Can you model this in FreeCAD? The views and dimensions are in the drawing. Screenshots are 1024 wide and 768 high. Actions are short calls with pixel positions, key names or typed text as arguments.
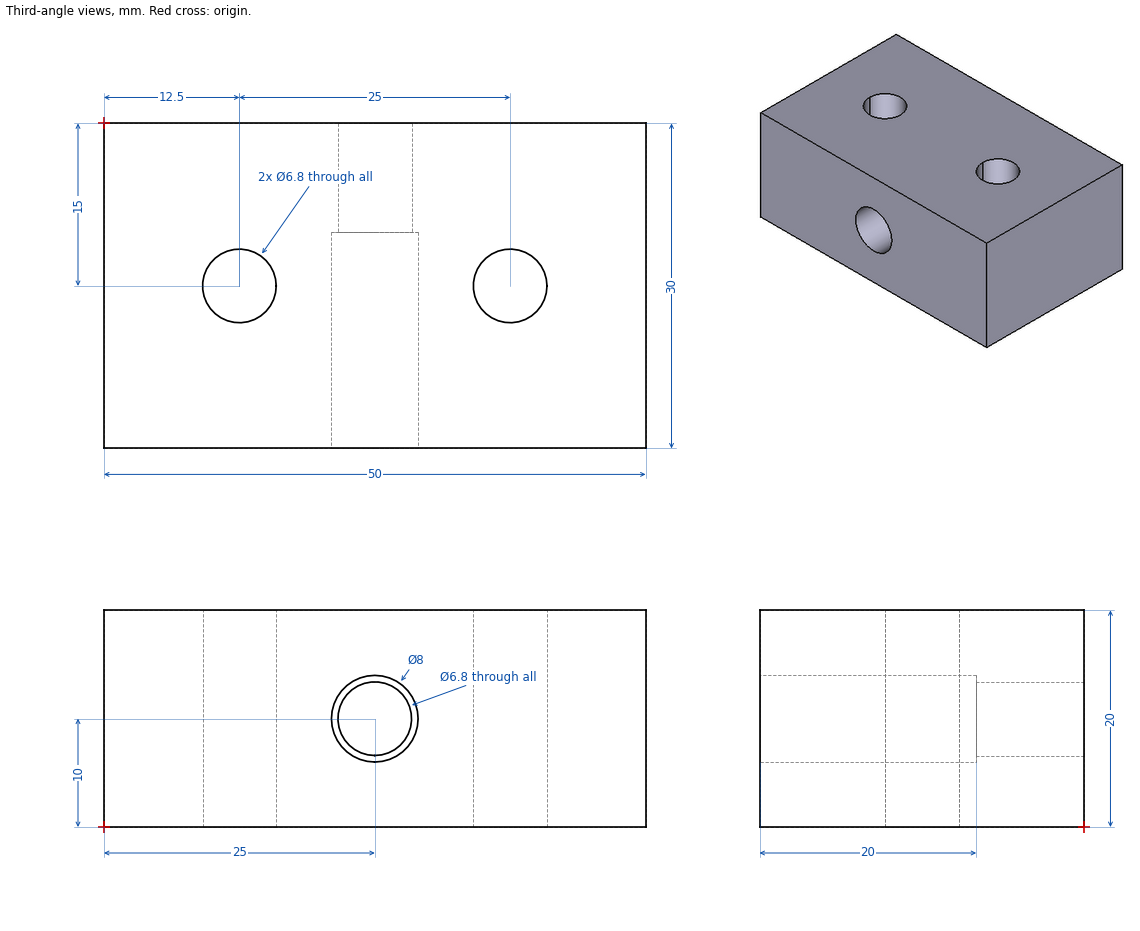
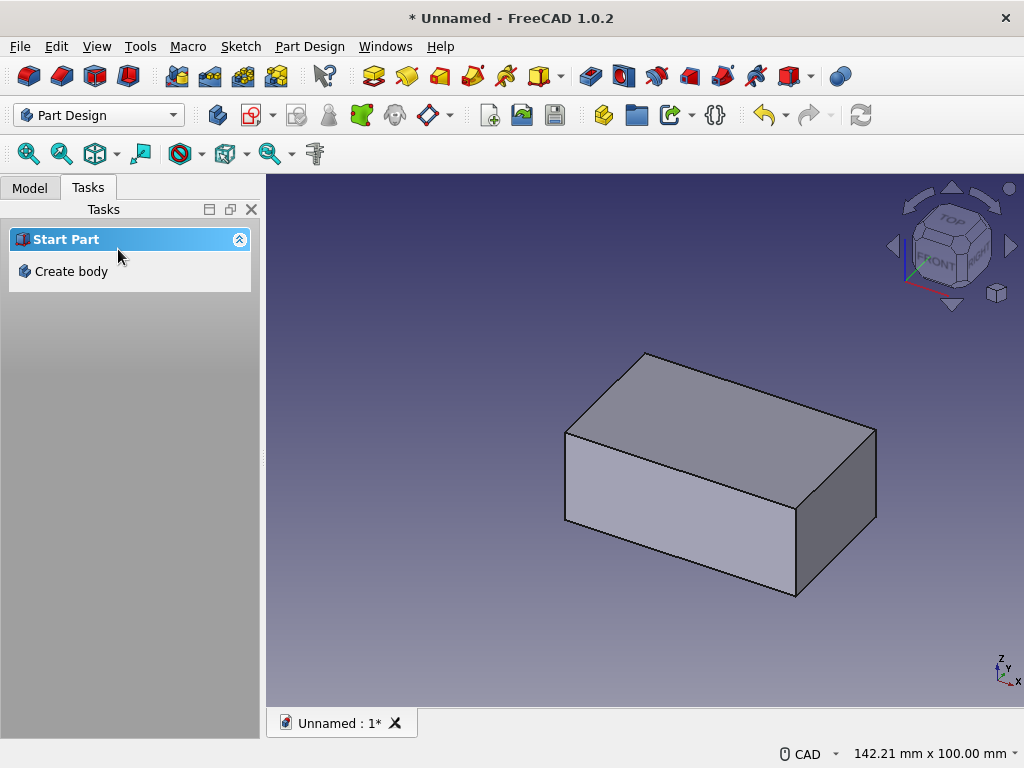
click(250, 116)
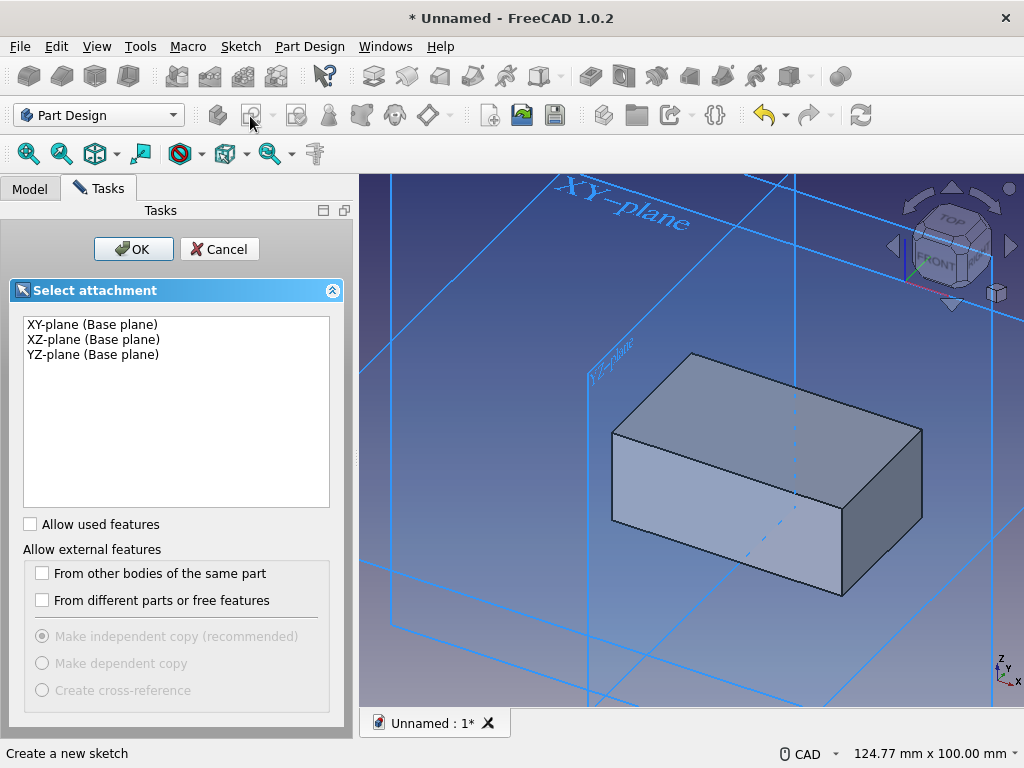
click(84, 324)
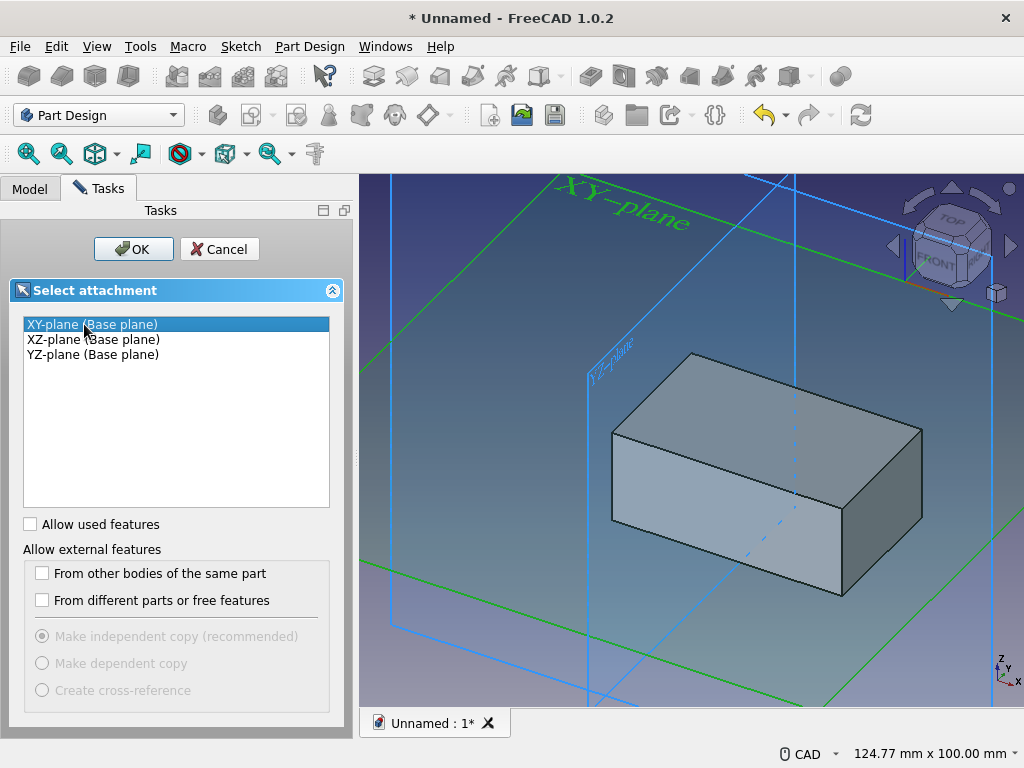
click(134, 249)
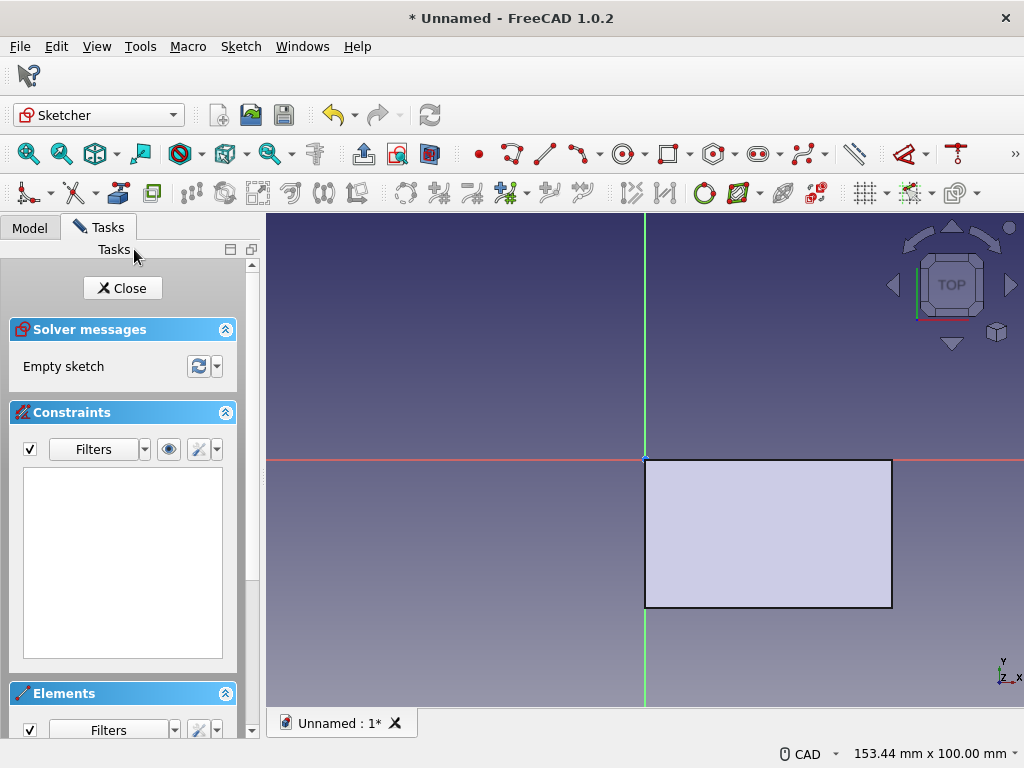
click(430, 154)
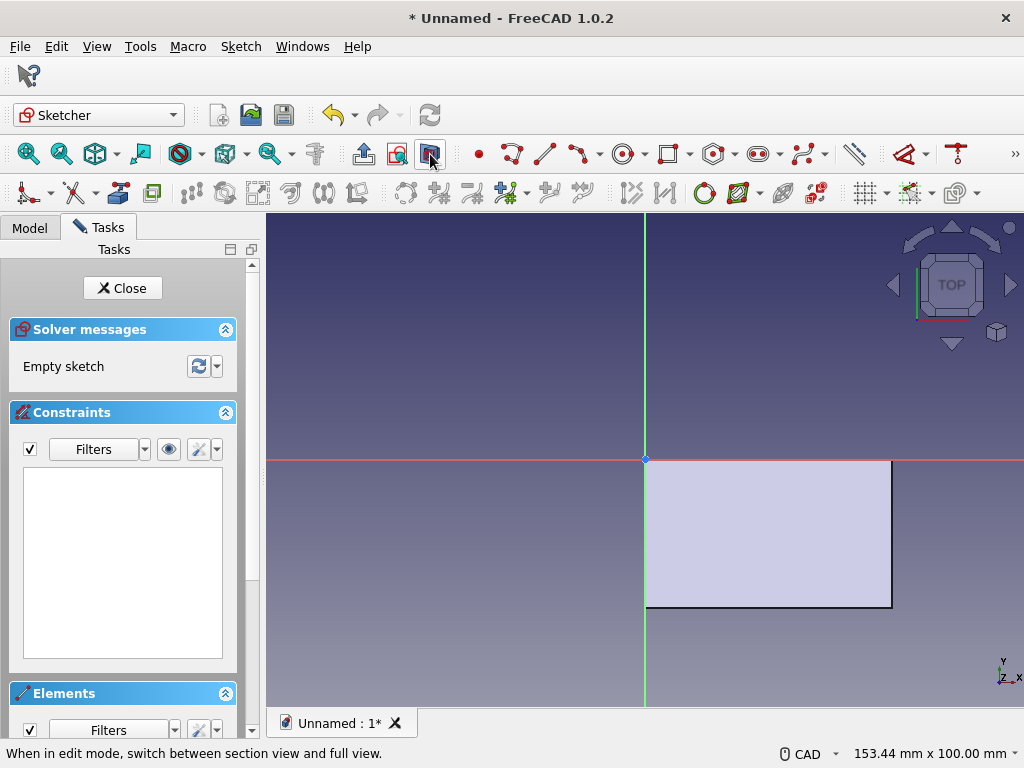
scroll(576, 460, down, 5)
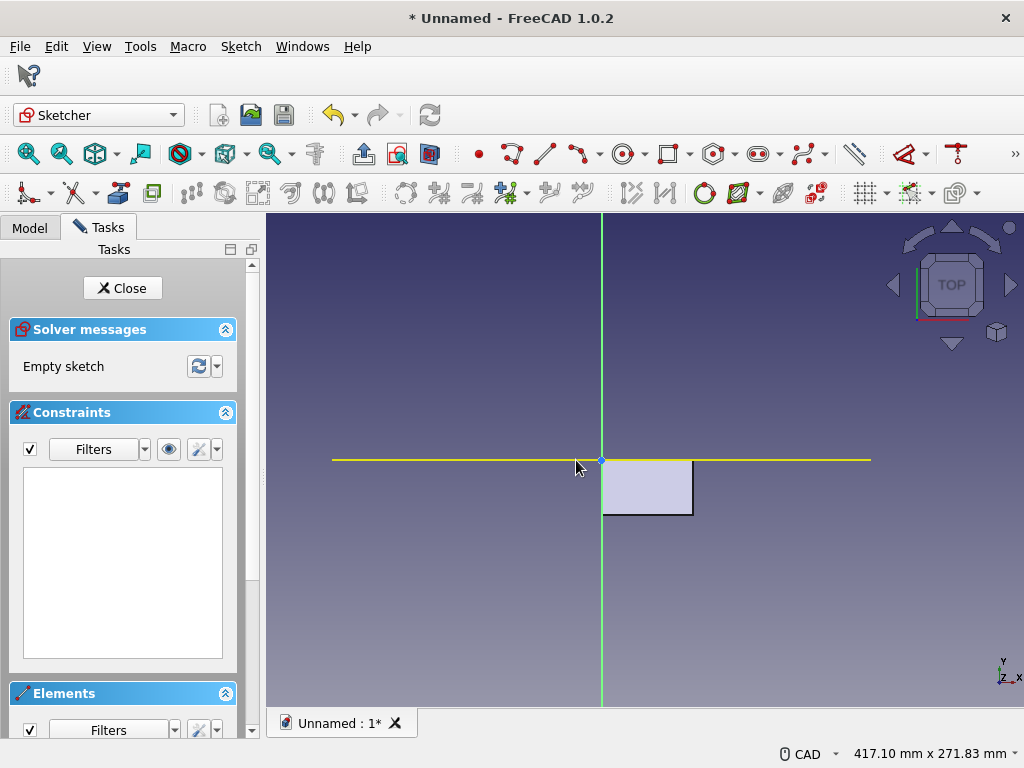
scroll(655, 481, up, 8)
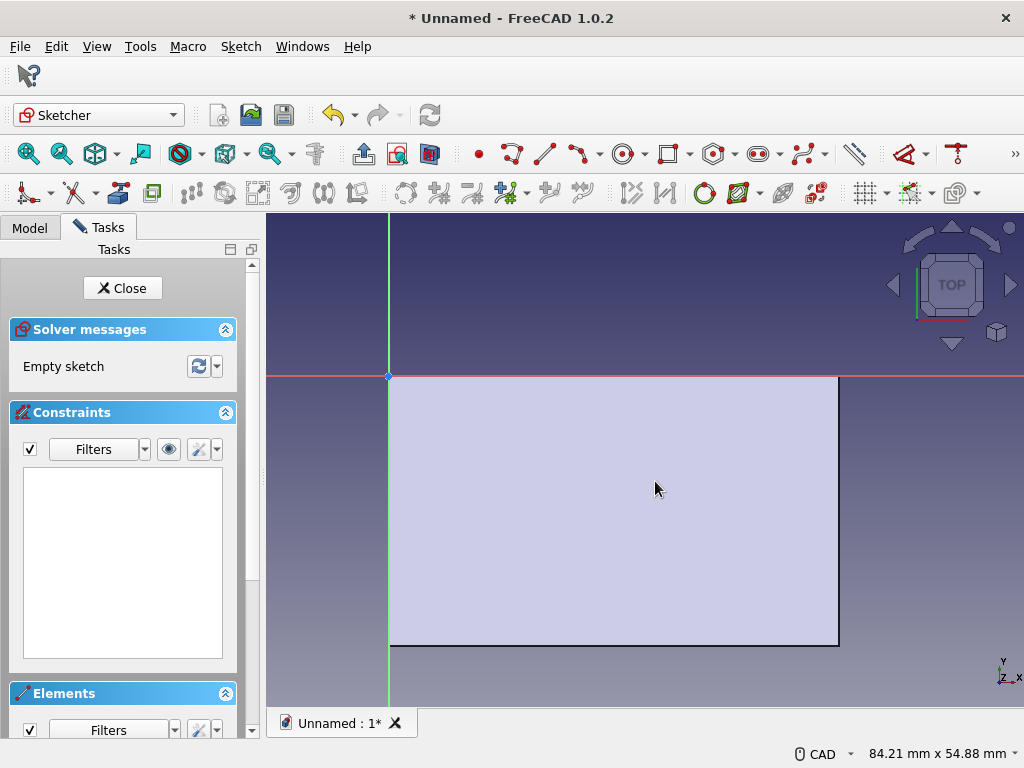
click(622, 154)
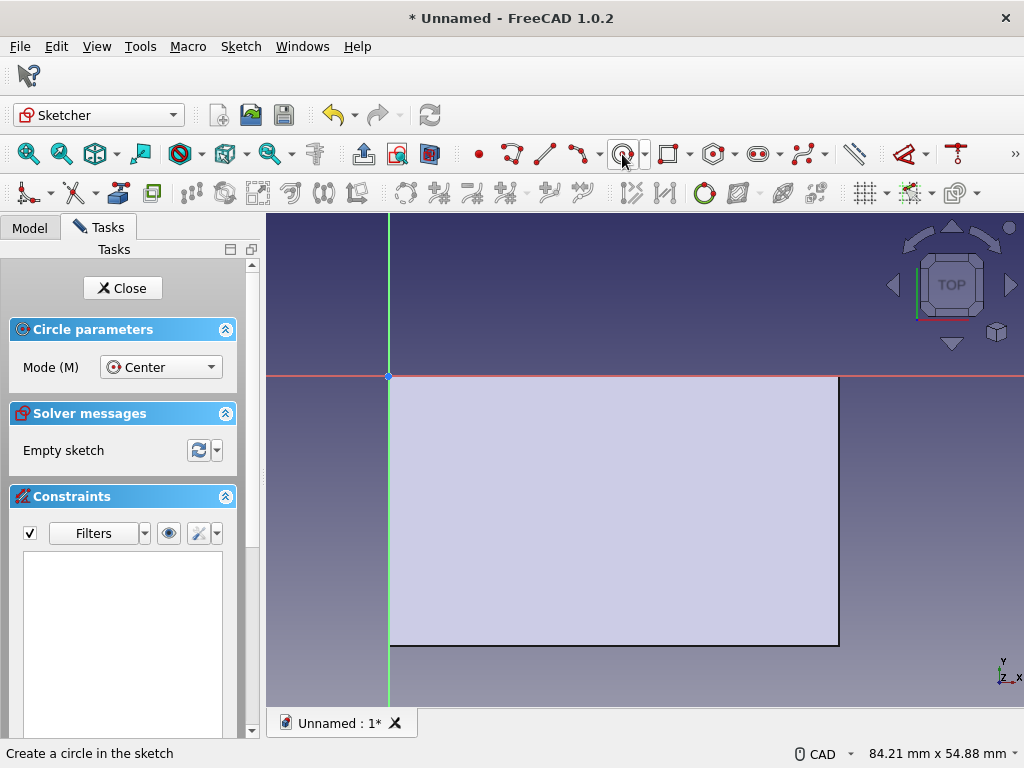
click(501, 511)
move(523, 490)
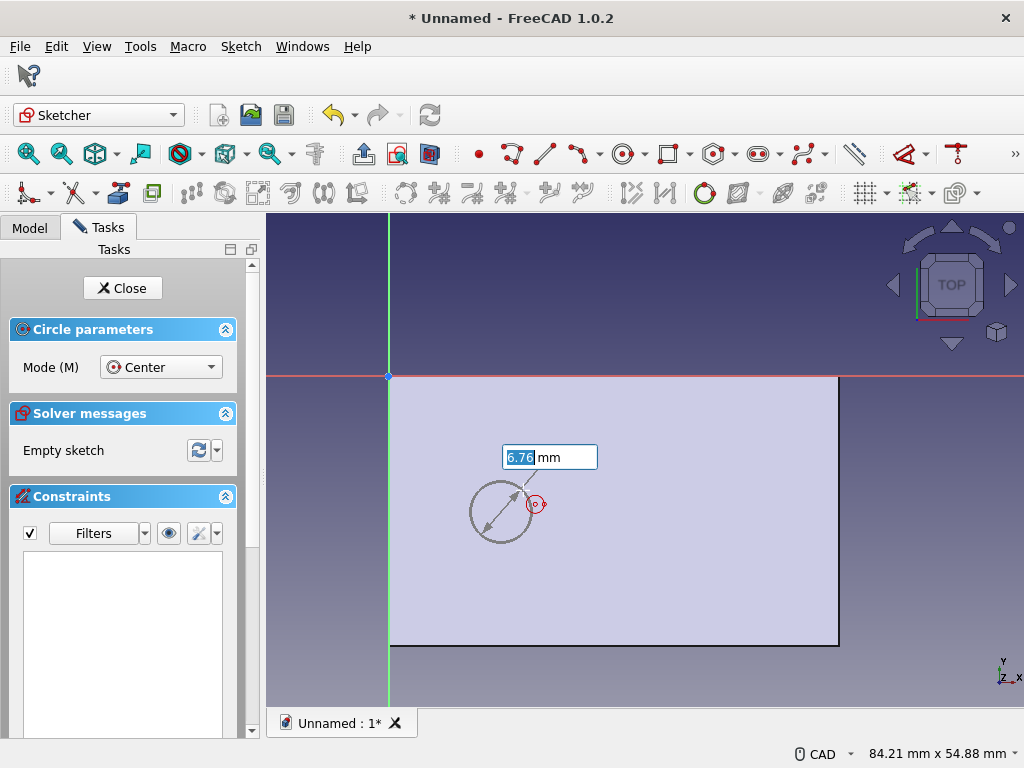
text(6.8)
key(Return)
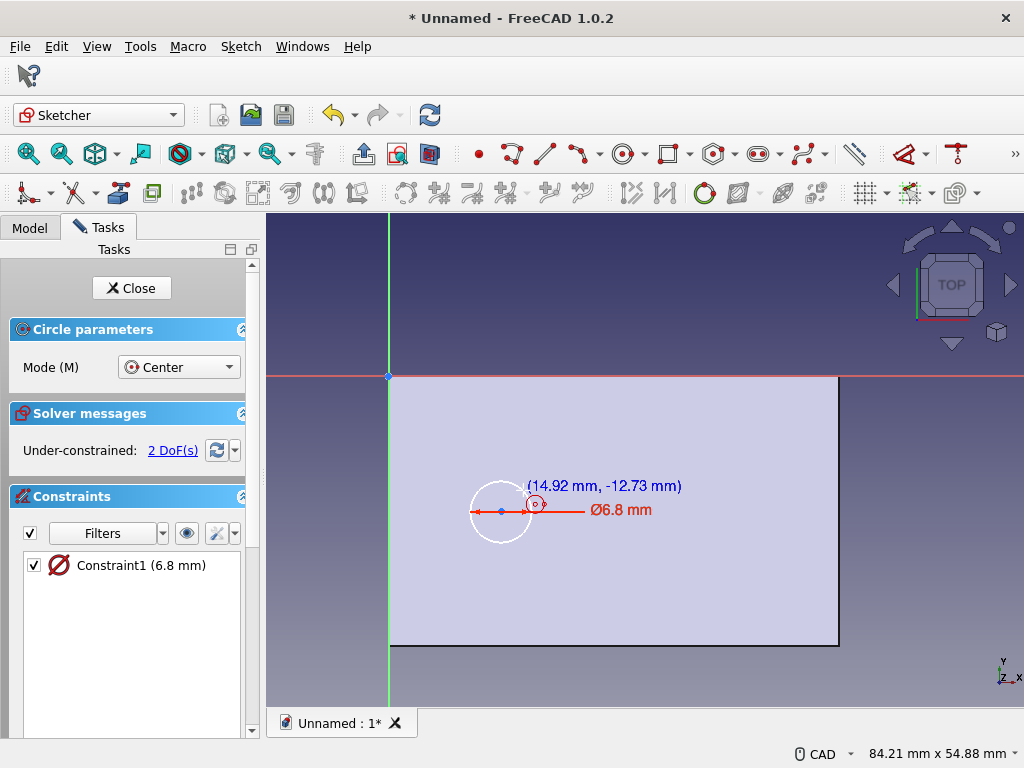
click(726, 511)
move(748, 490)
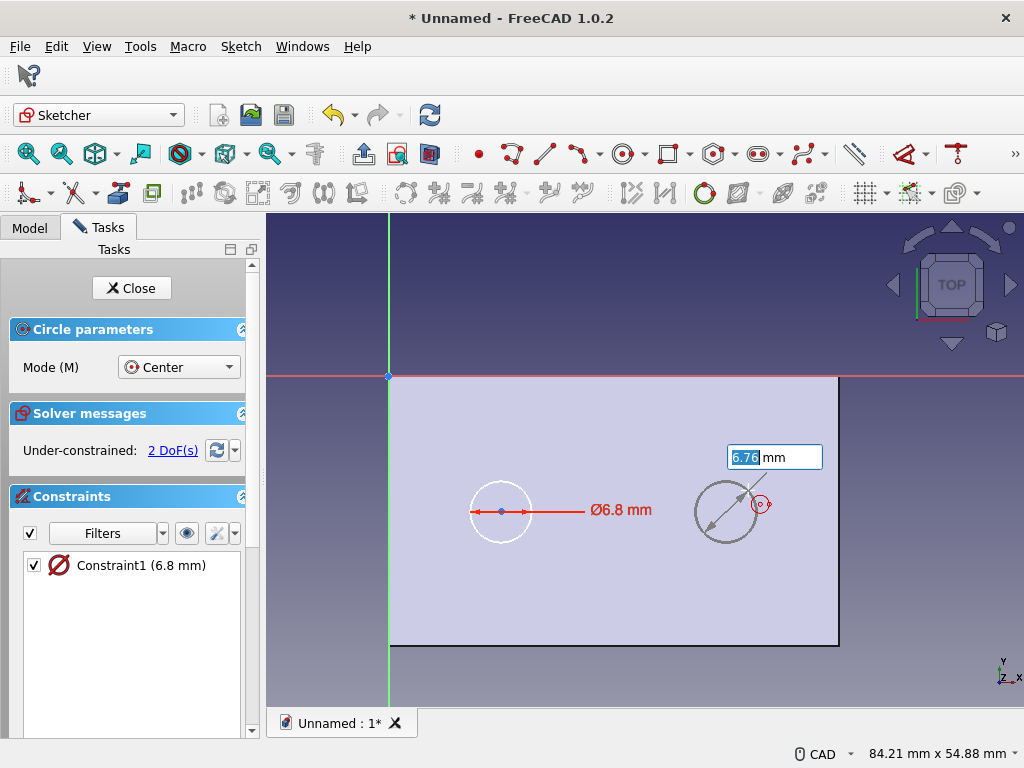
text(6.8)
key(Return)
key(Escape)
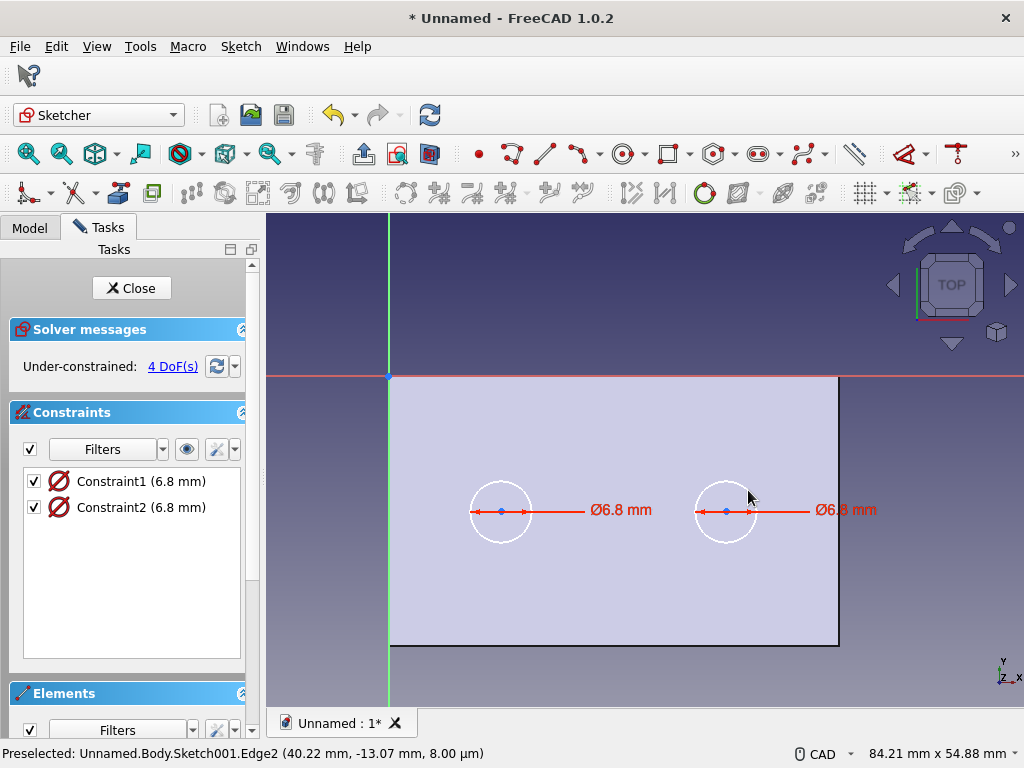
click(501, 512)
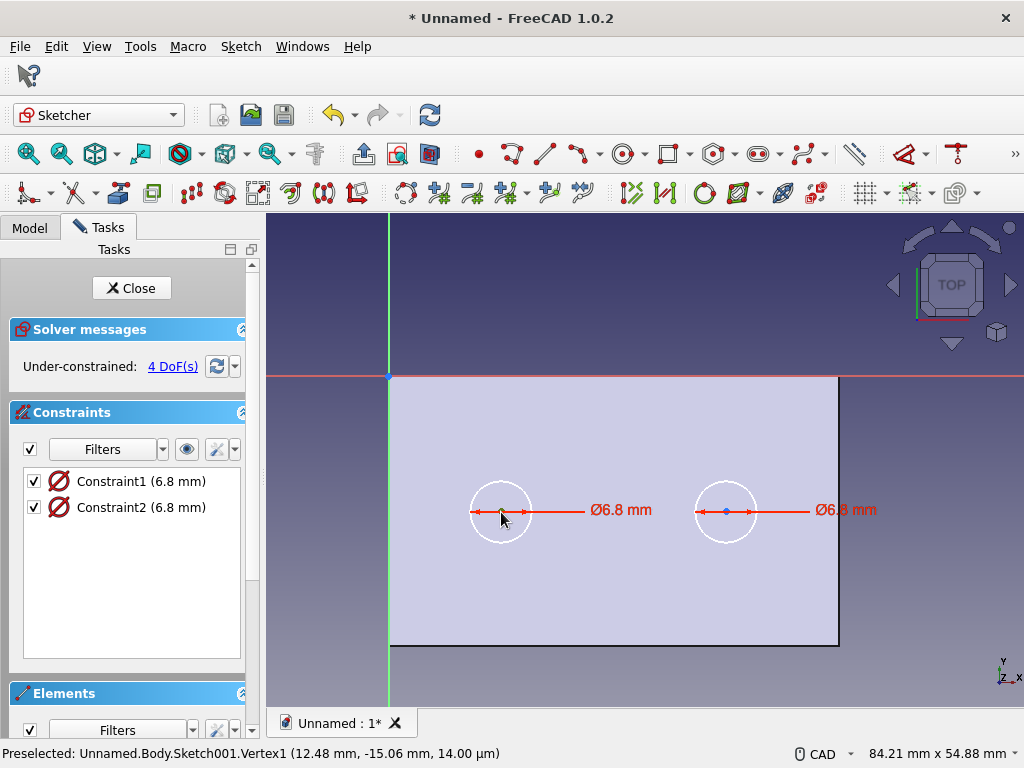
click(726, 512)